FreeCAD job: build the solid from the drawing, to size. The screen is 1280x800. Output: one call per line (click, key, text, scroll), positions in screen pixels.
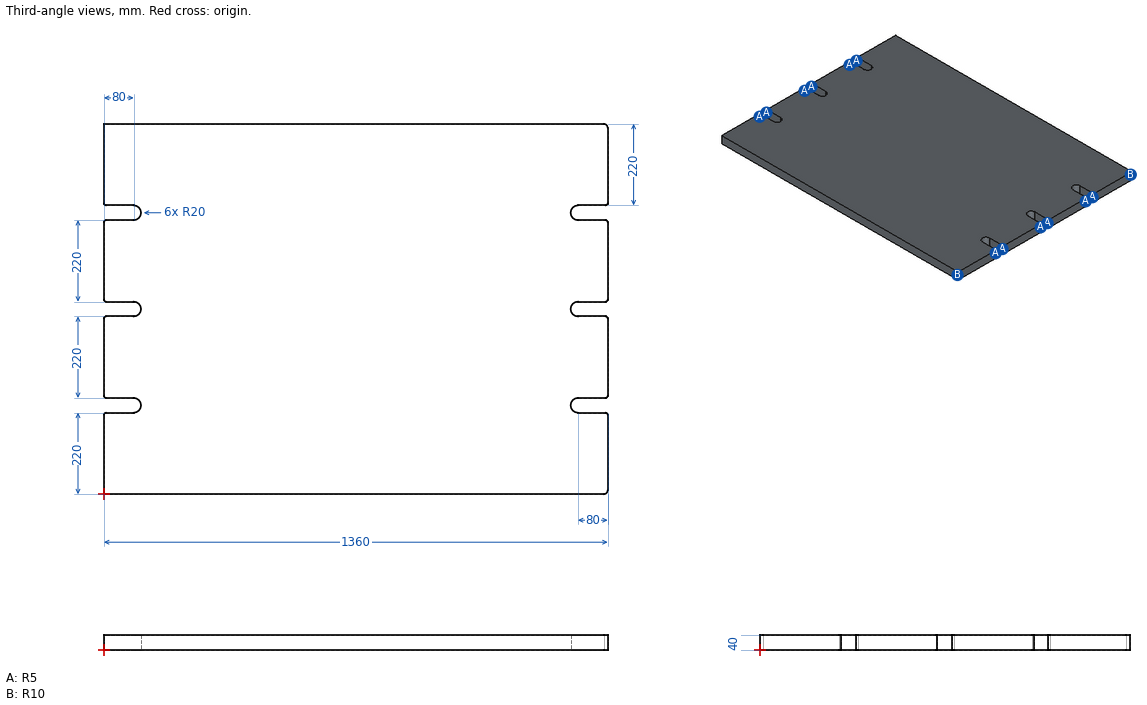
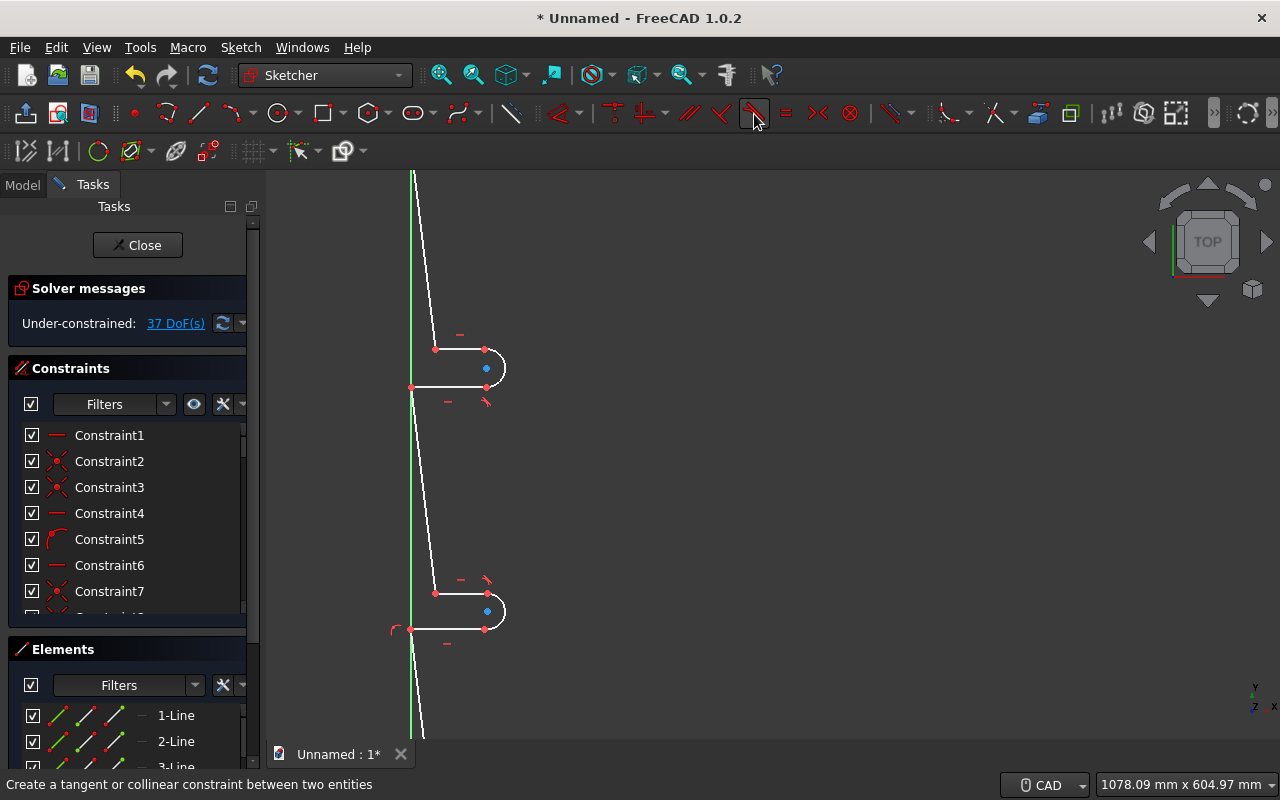
click(462, 629)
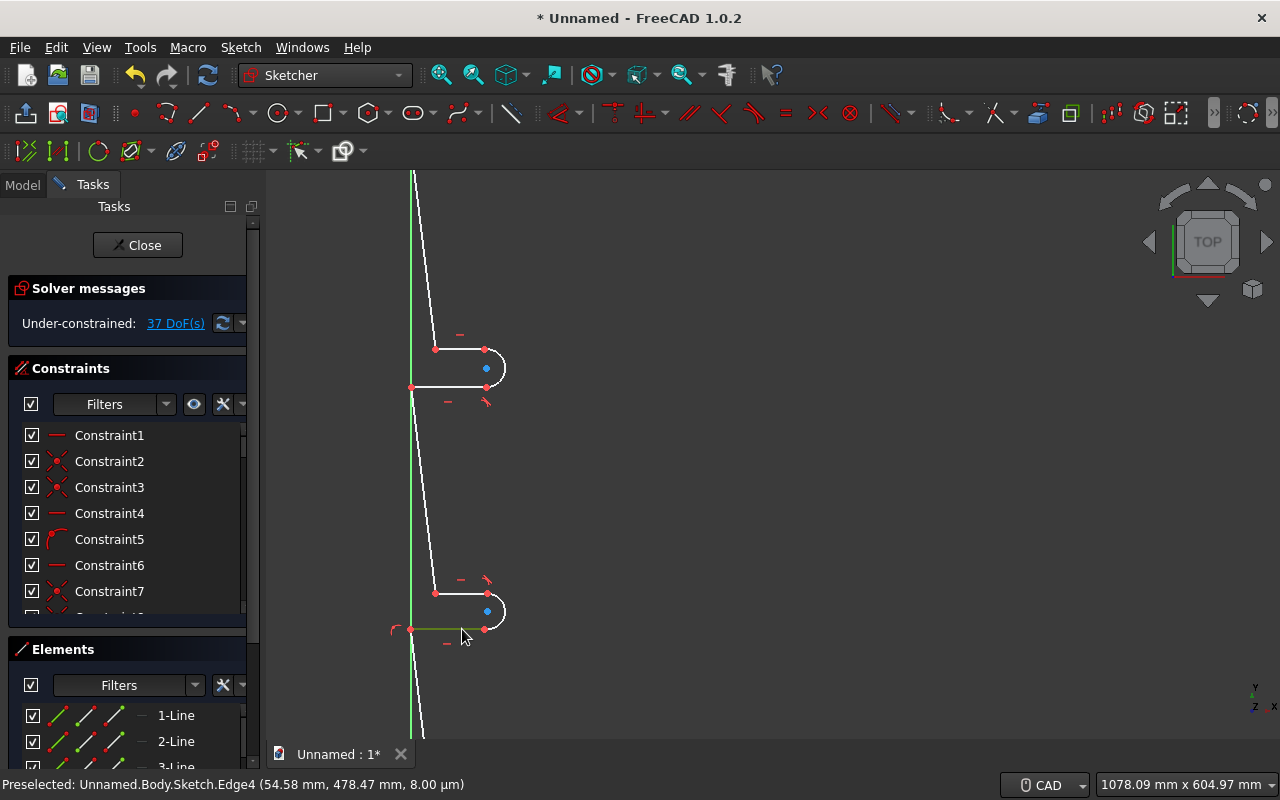
click(500, 623)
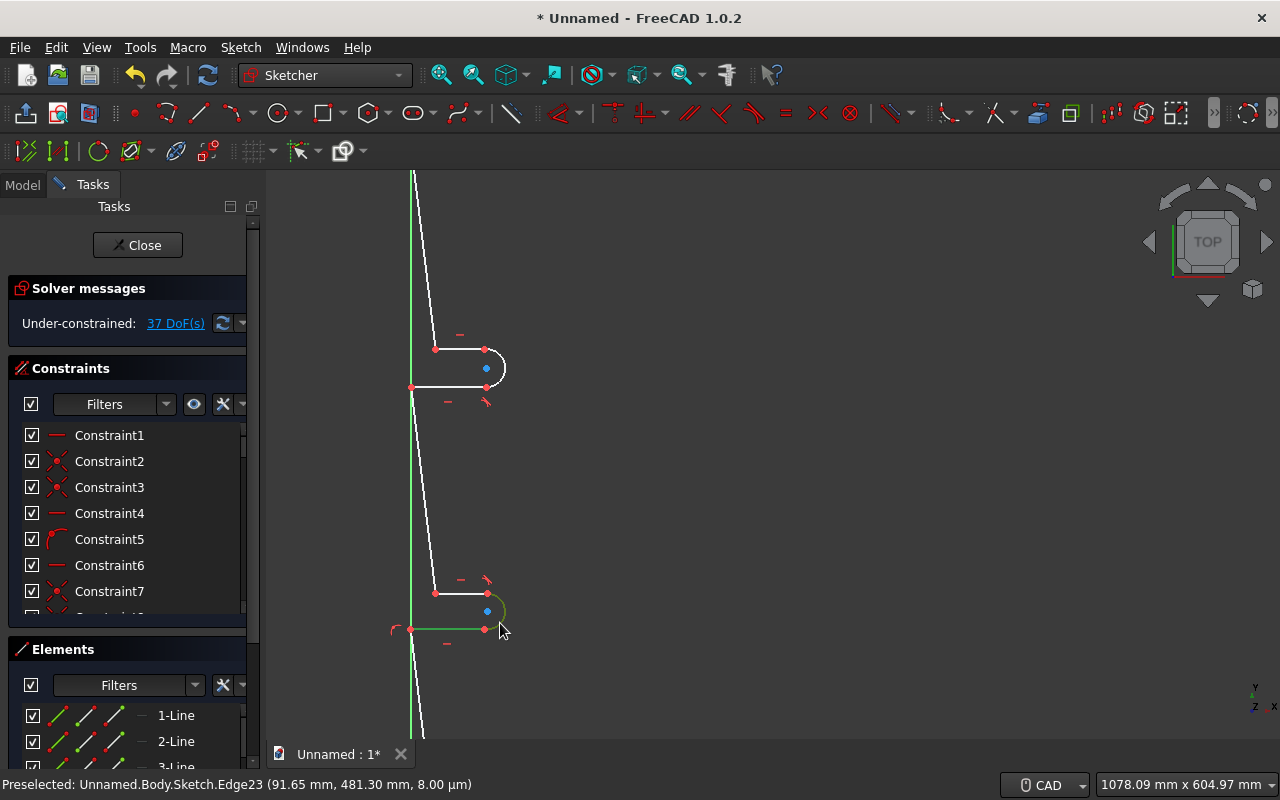
click(754, 114)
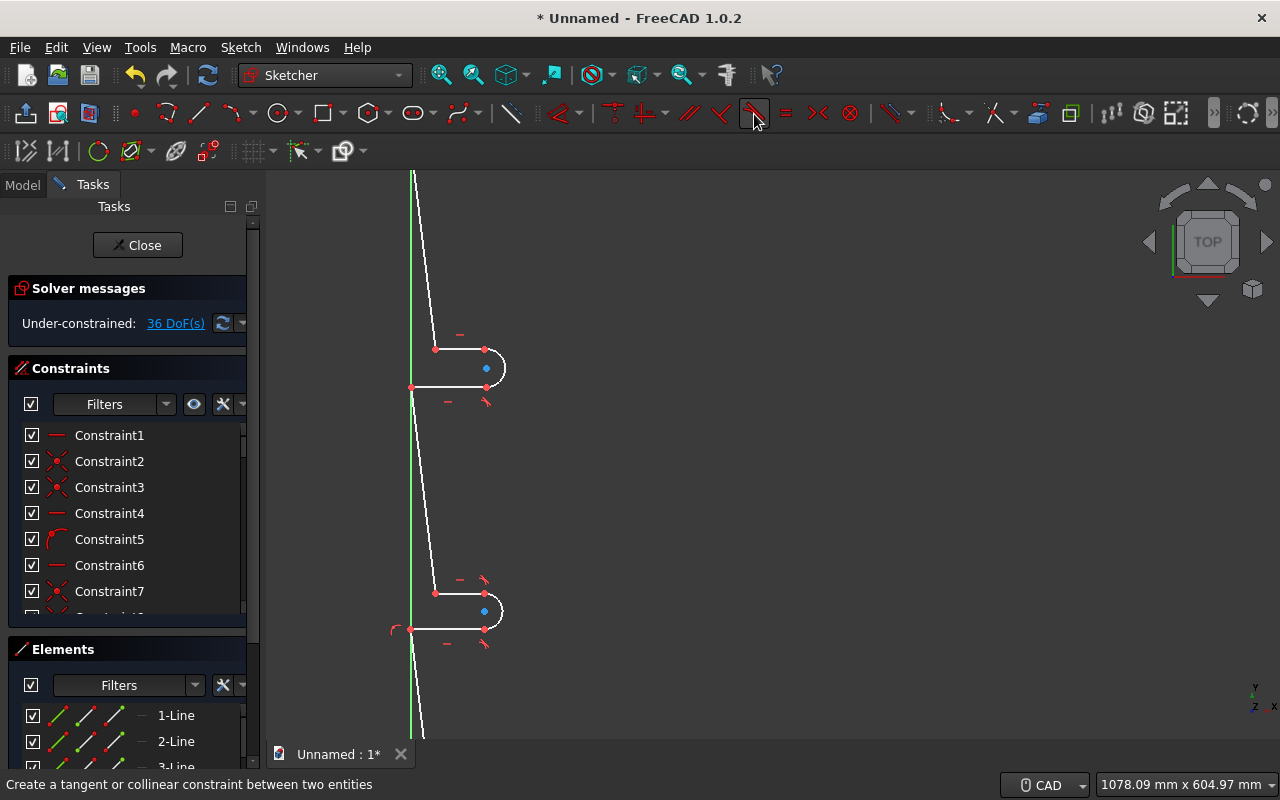
scroll(503, 365, down, 5)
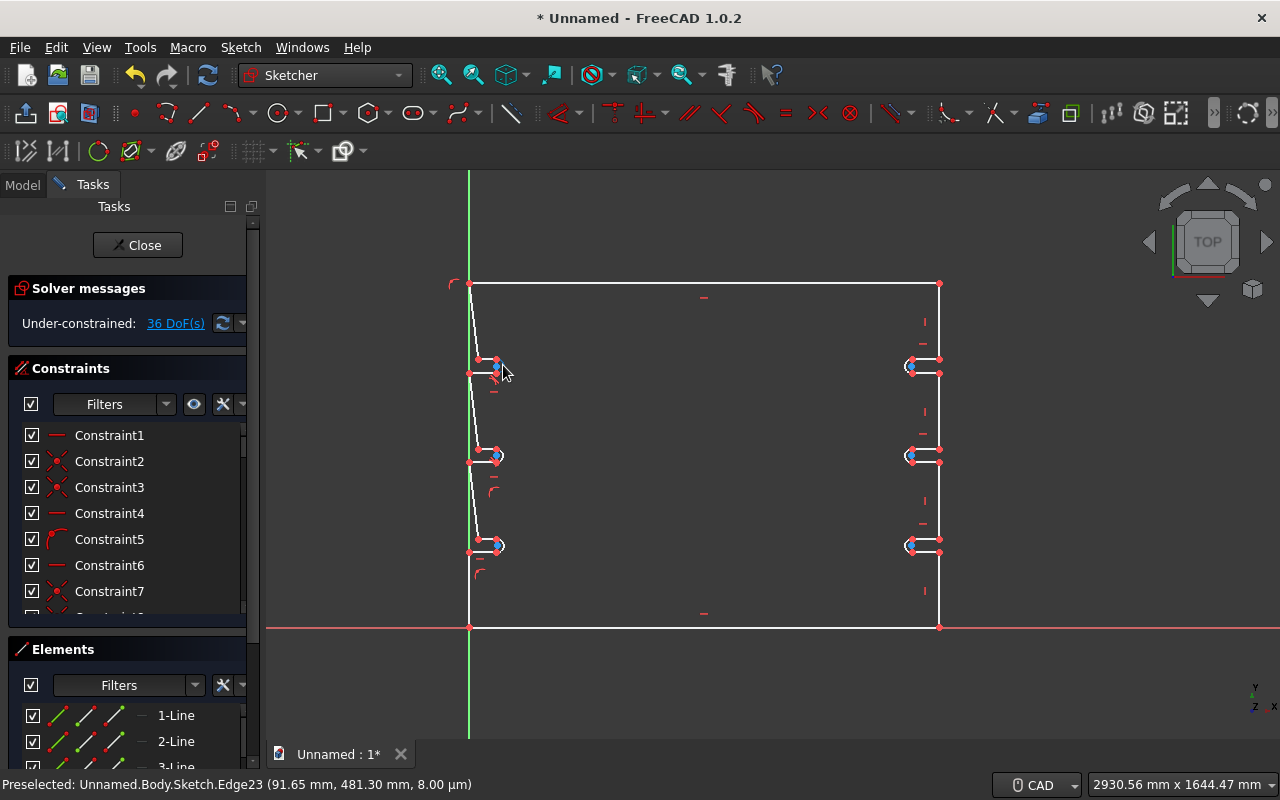
scroll(484, 539, up, 5)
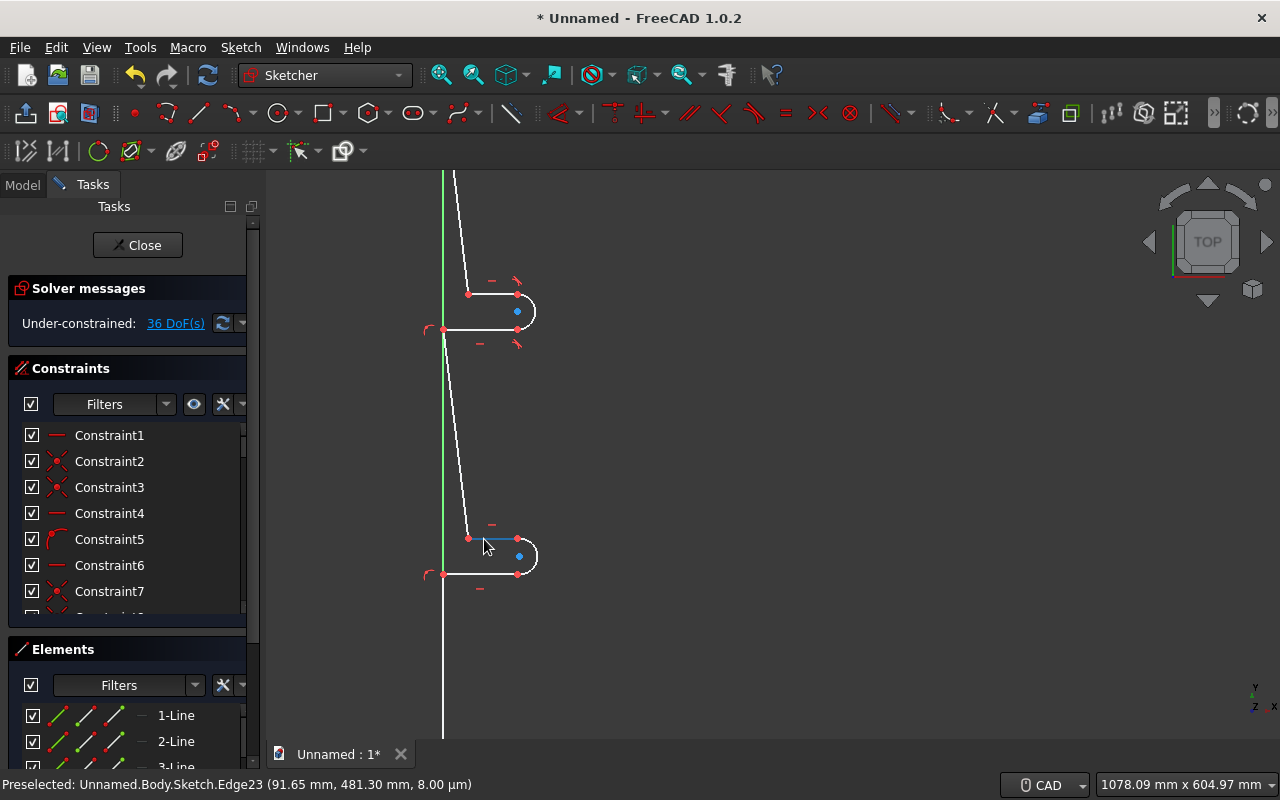
click(483, 539)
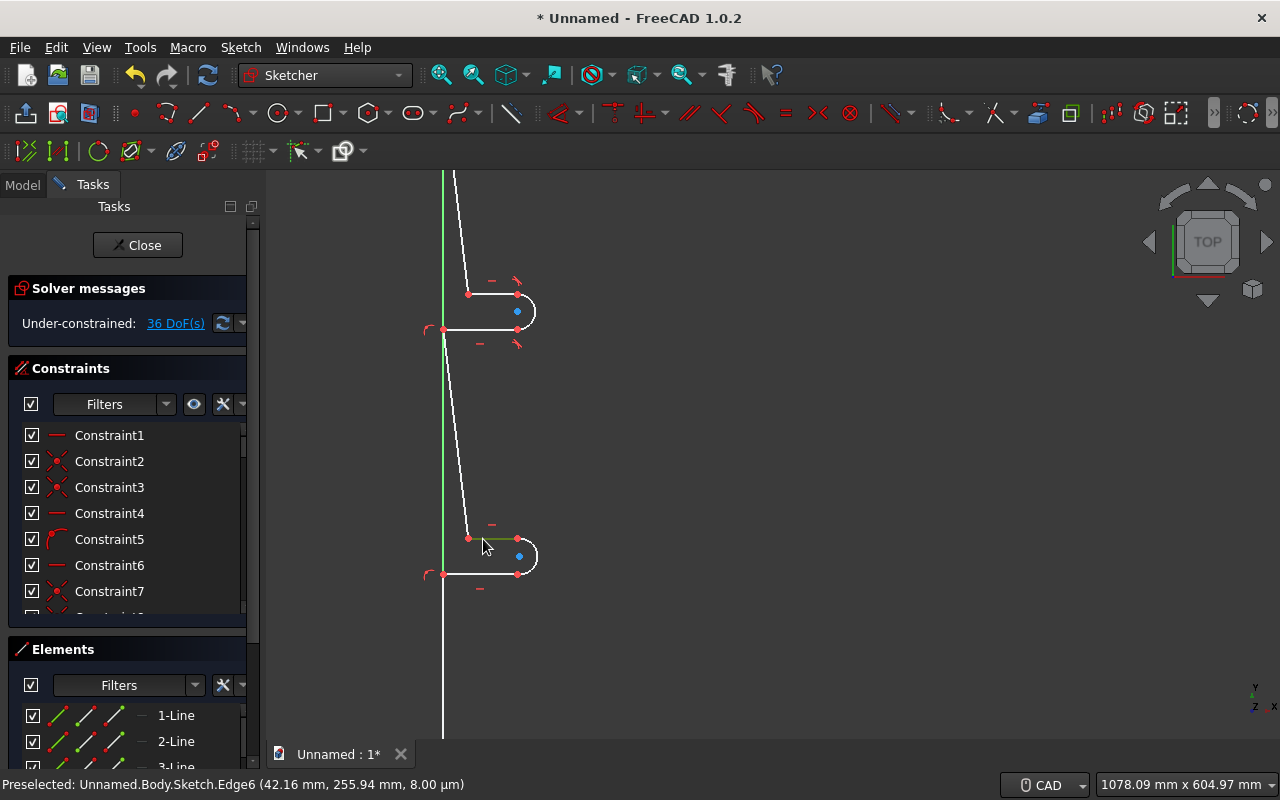
click(533, 568)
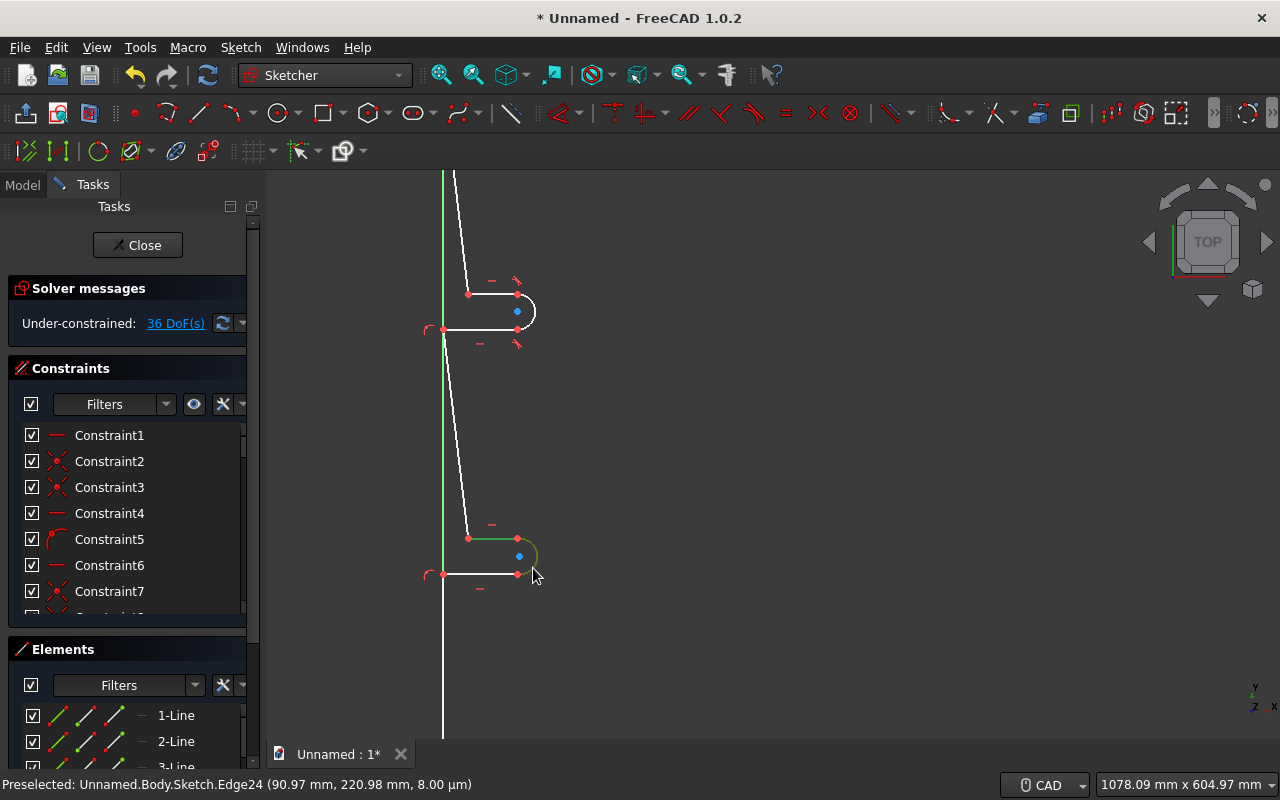
click(754, 114)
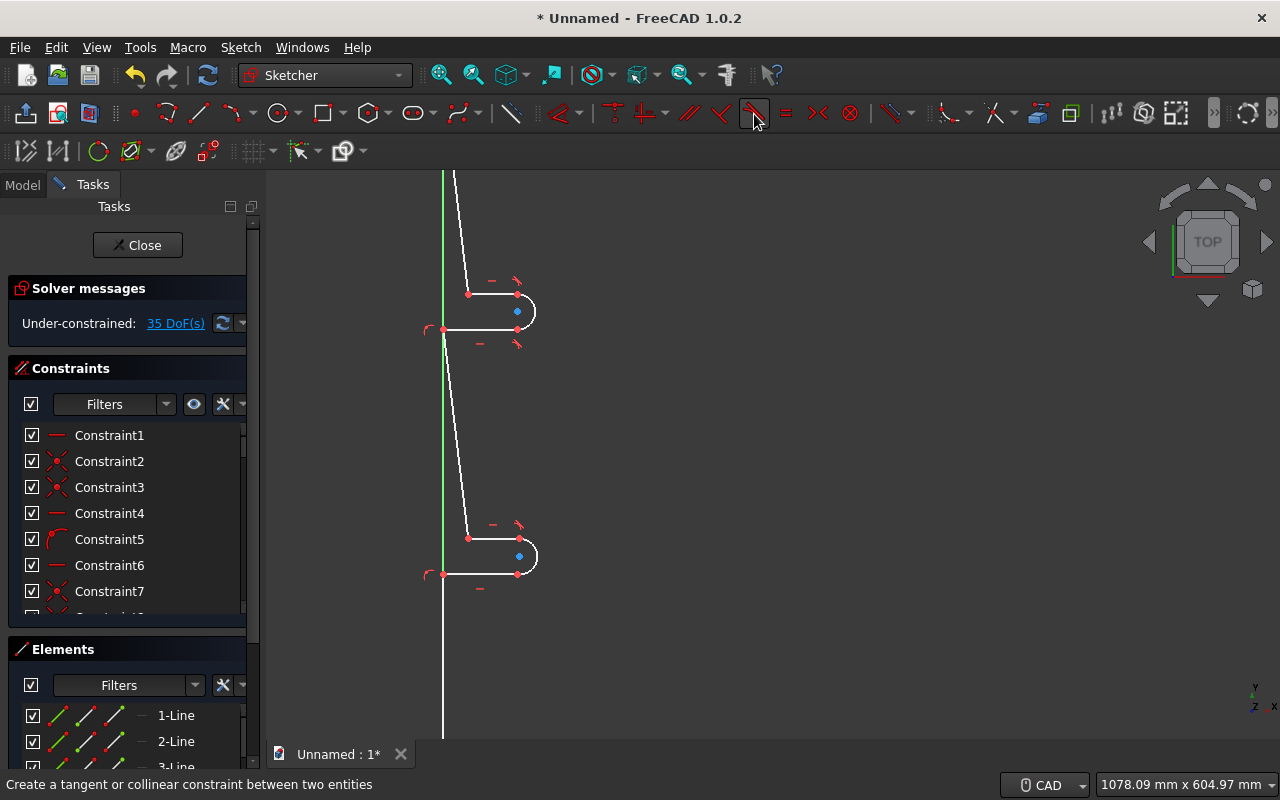
click(495, 574)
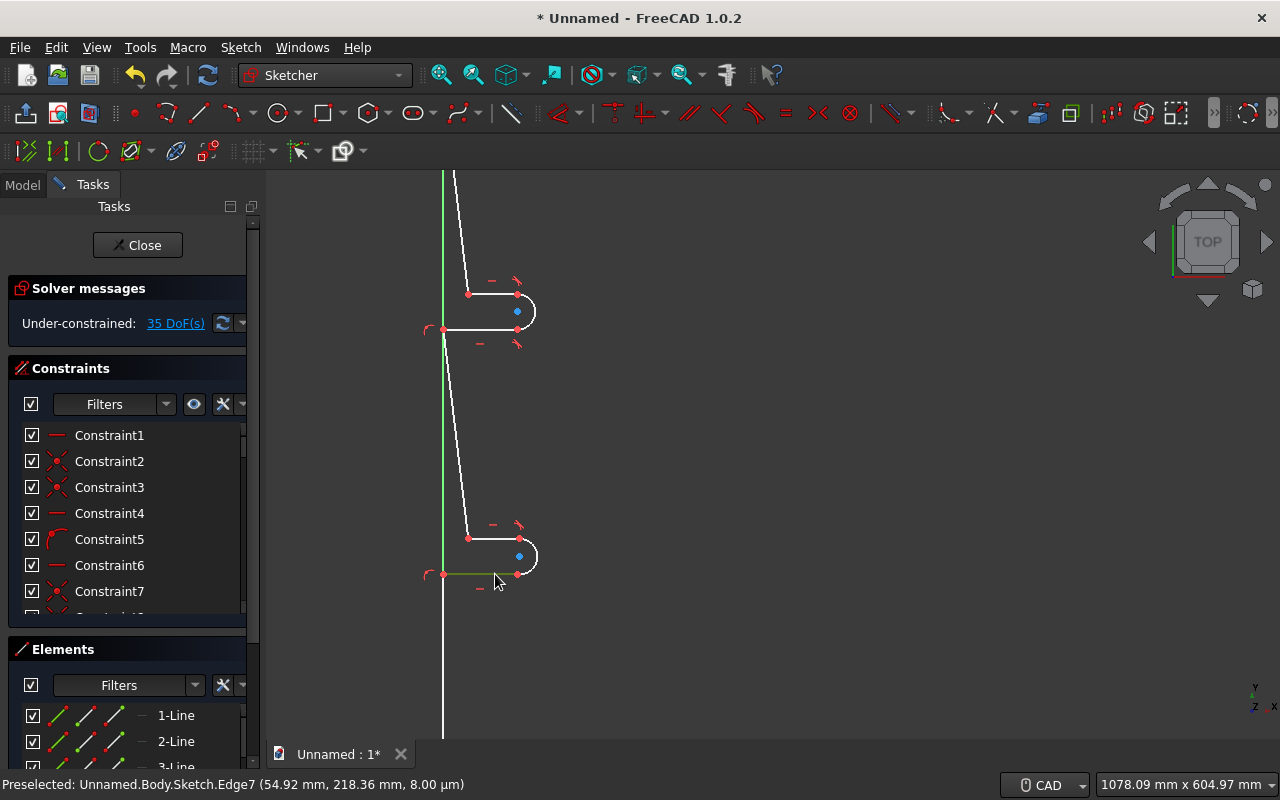
click(533, 568)